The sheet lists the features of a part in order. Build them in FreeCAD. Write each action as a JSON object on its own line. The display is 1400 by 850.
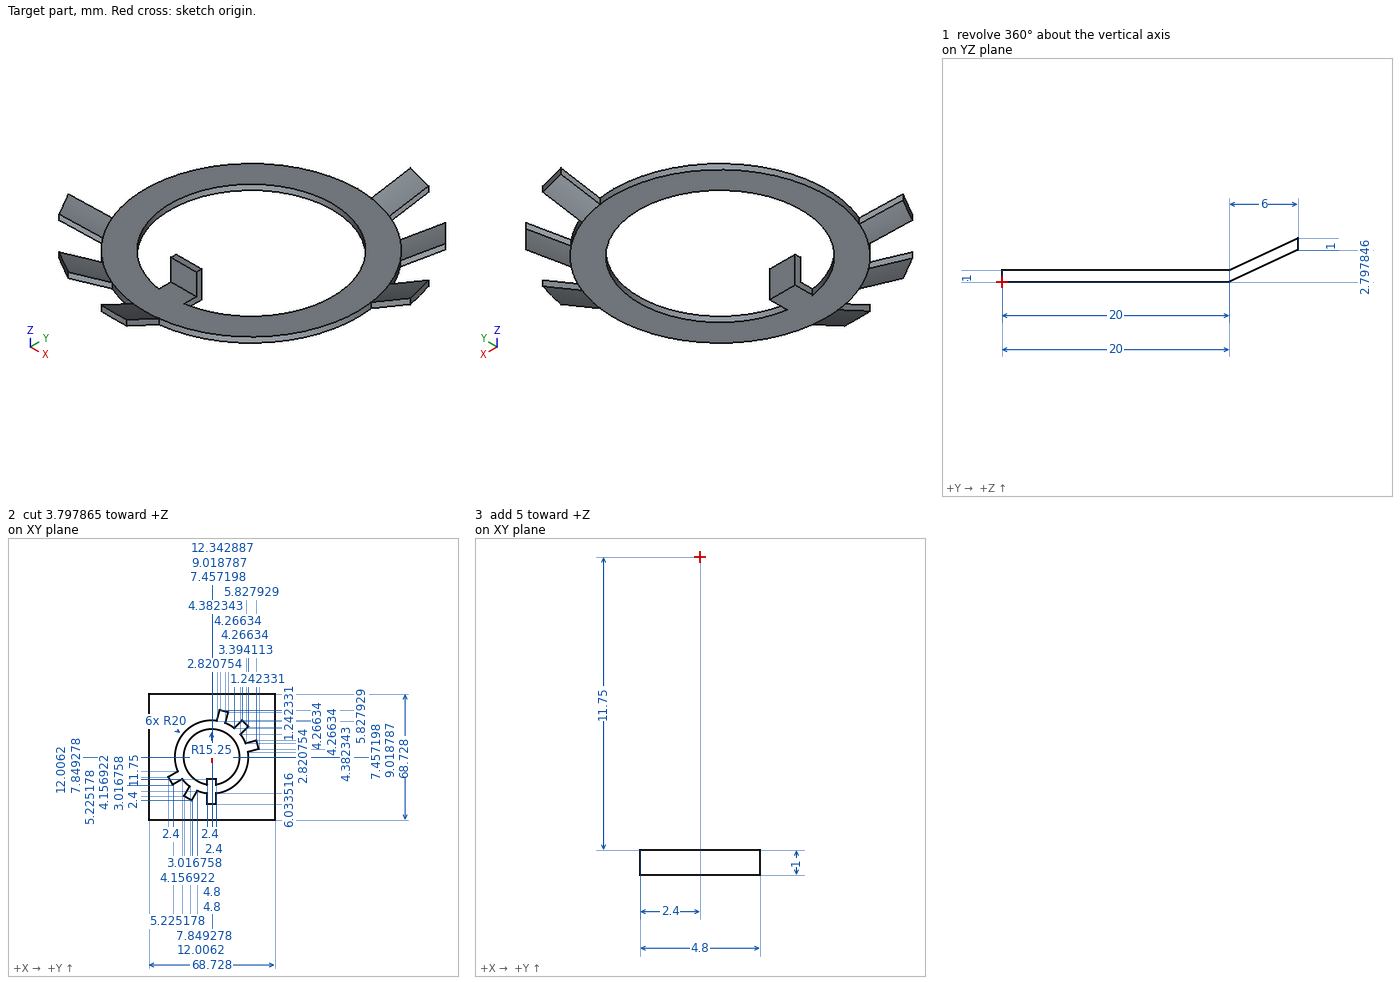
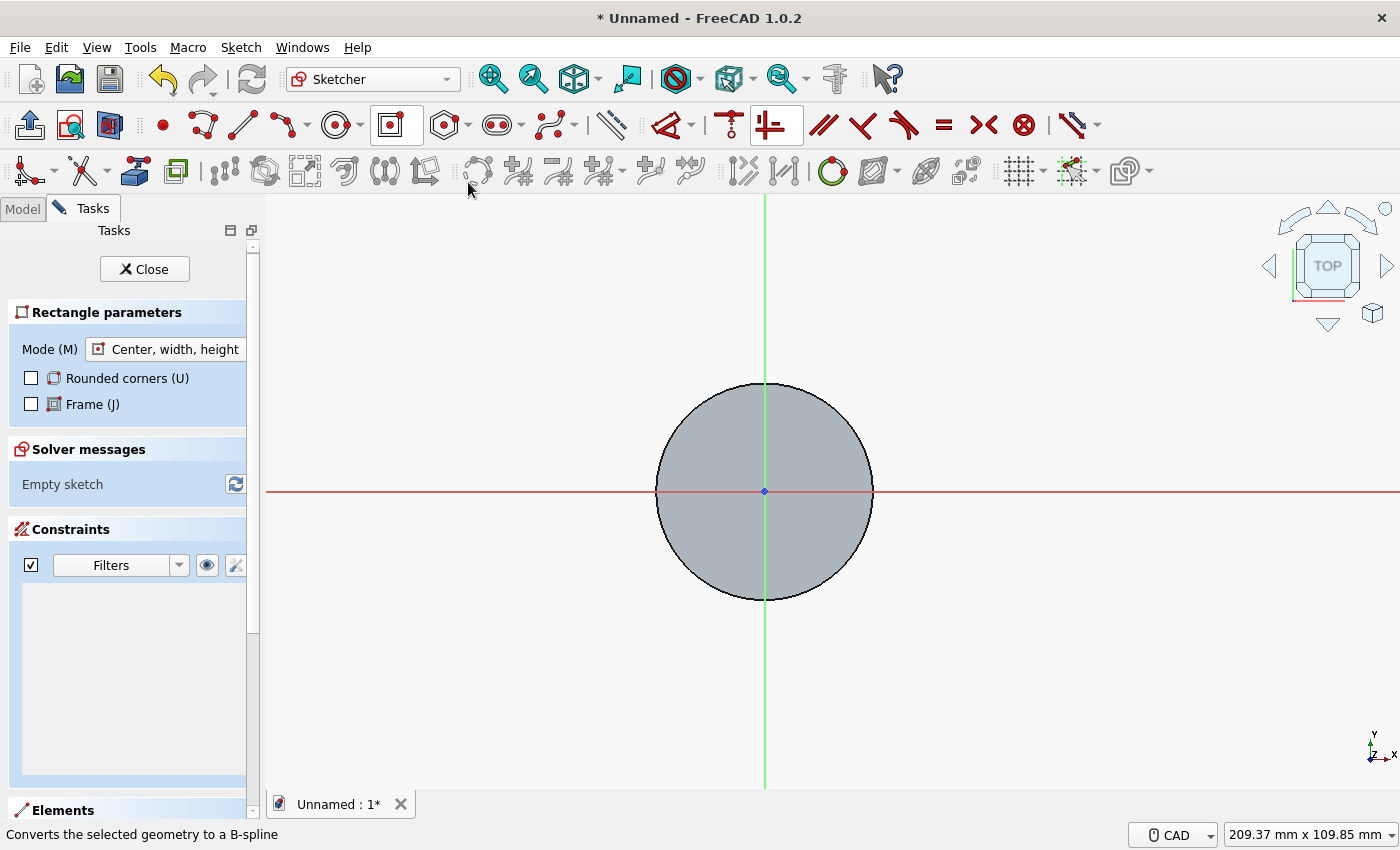
{"action": "left_click", "coordinate": [765, 492]}
{"action": "mouse_move", "coordinate": [951, 306]}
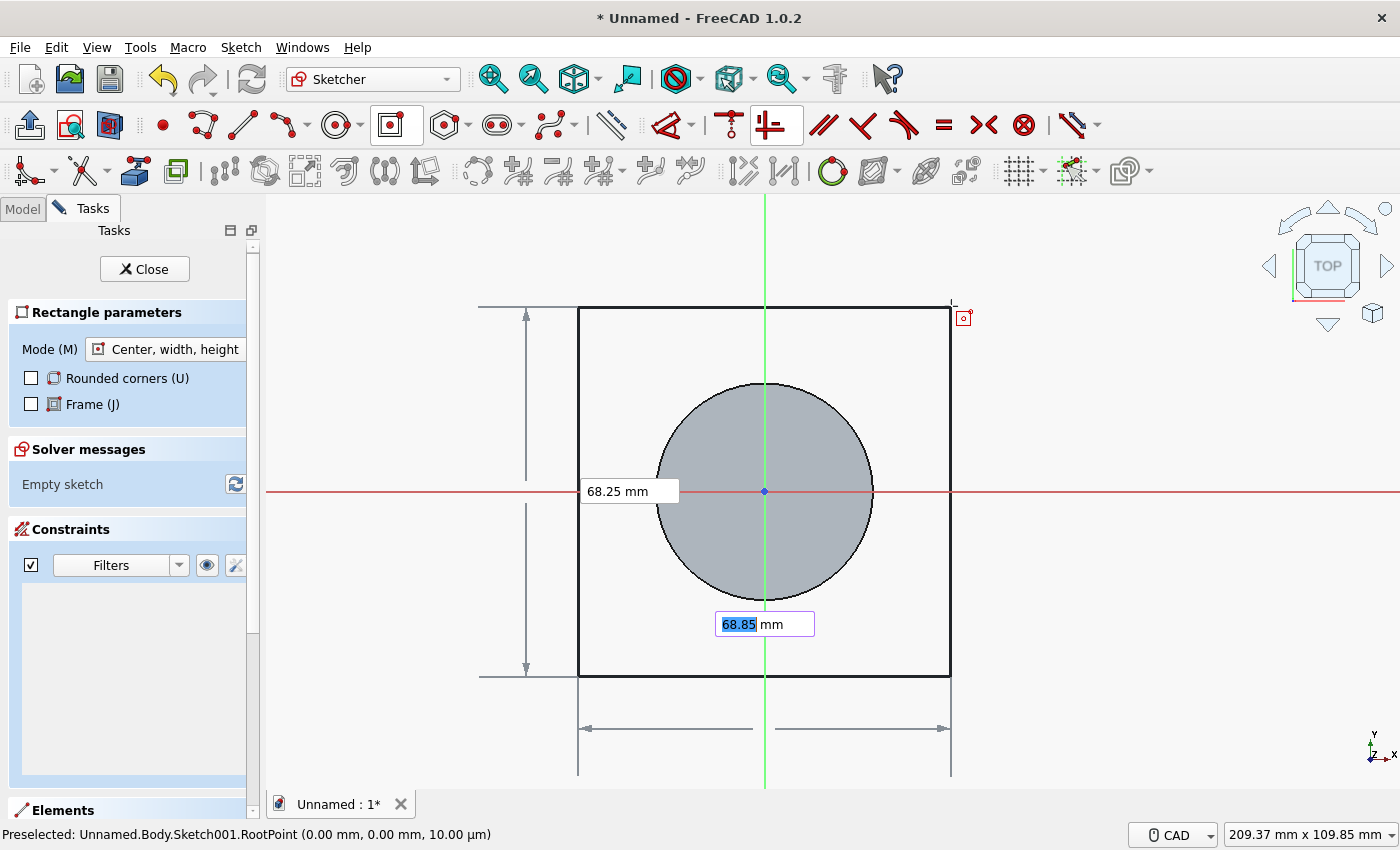
{"action": "type", "text": "68.728"}
{"action": "key", "text": "Tab"}
{"action": "type", "text": "68.728"}
{"action": "key", "text": "Return"}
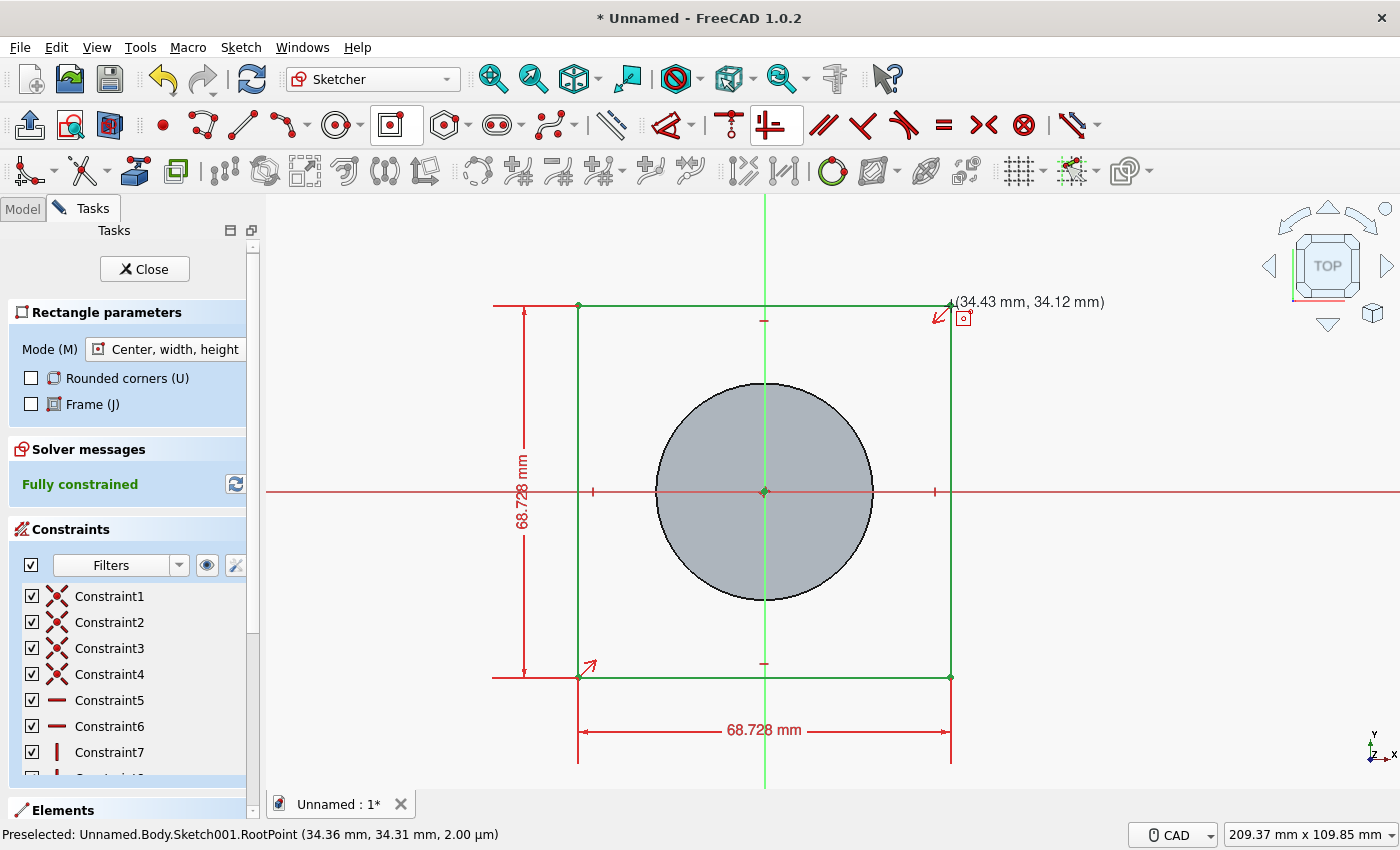
{"action": "left_click", "coordinate": [204, 126]}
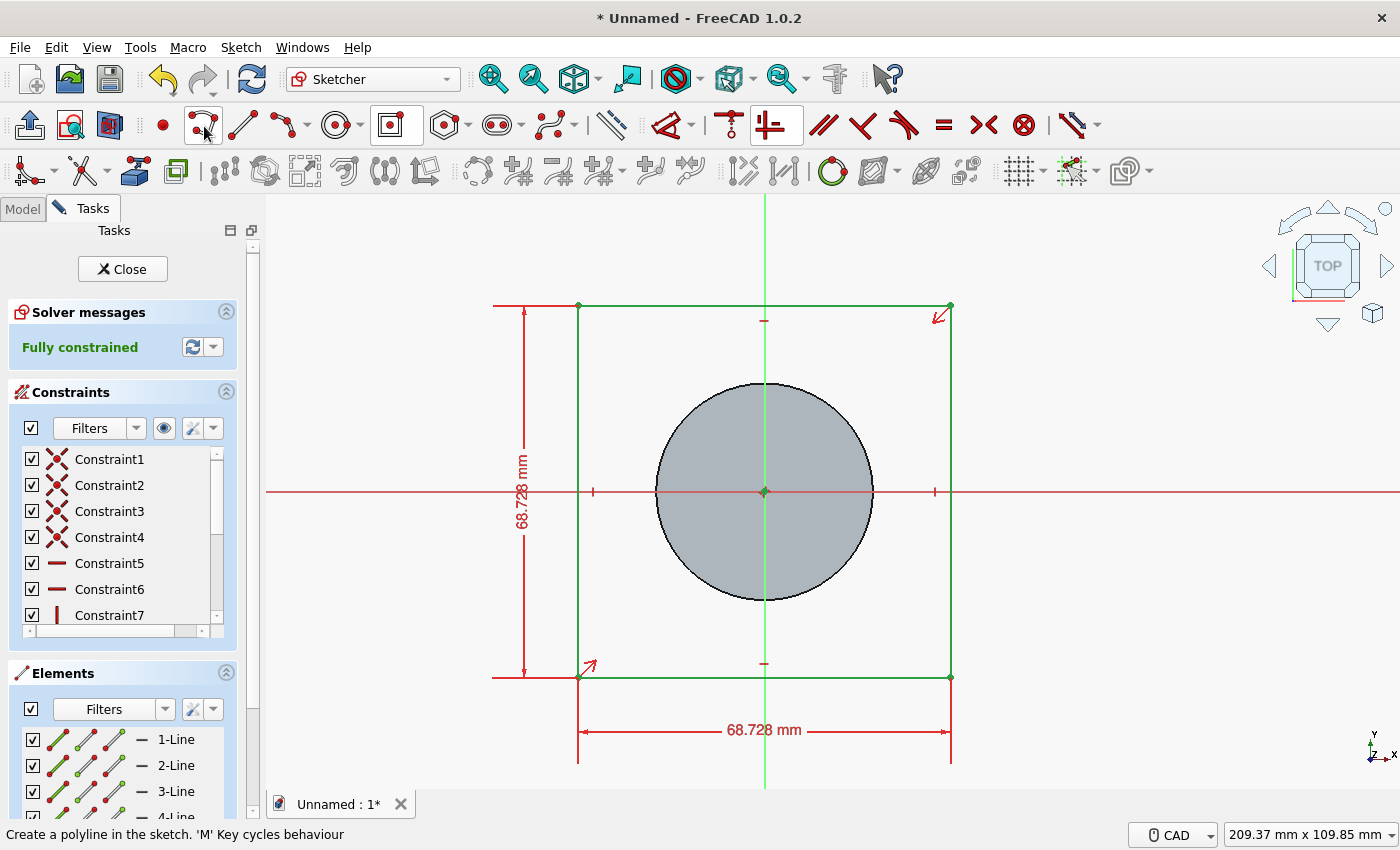
{"action": "scroll", "coordinate": [752, 573], "scroll_direction": "up", "scroll_amount": 2}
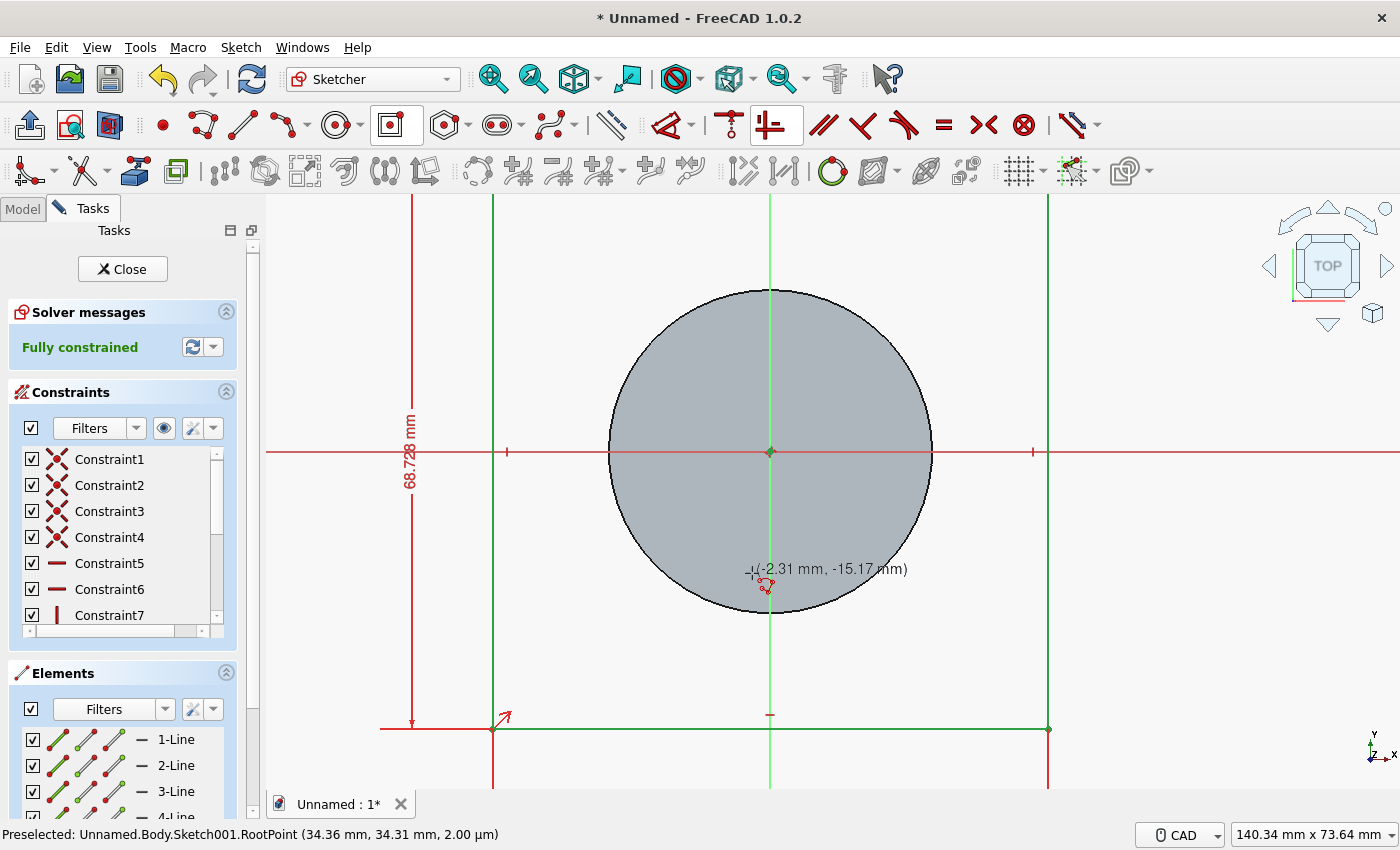
{"action": "left_click", "coordinate": [751, 573]}
{"action": "left_click", "coordinate": [751, 547]}
{"action": "left_click", "coordinate": [790, 547]}
{"action": "left_click", "coordinate": [790, 573]}
{"action": "right_click", "coordinate": [790, 573]}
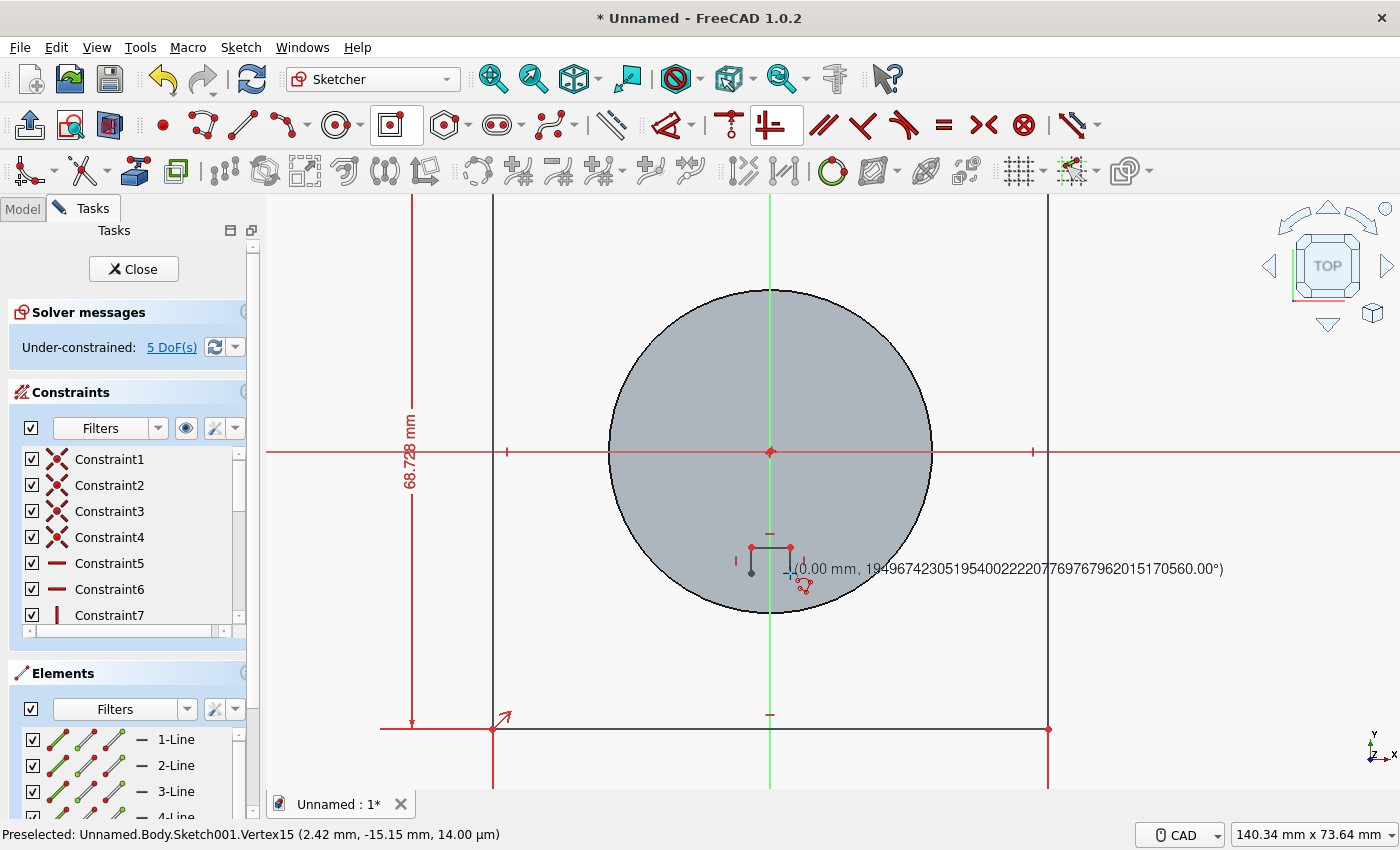
{"action": "left_click", "coordinate": [284, 126]}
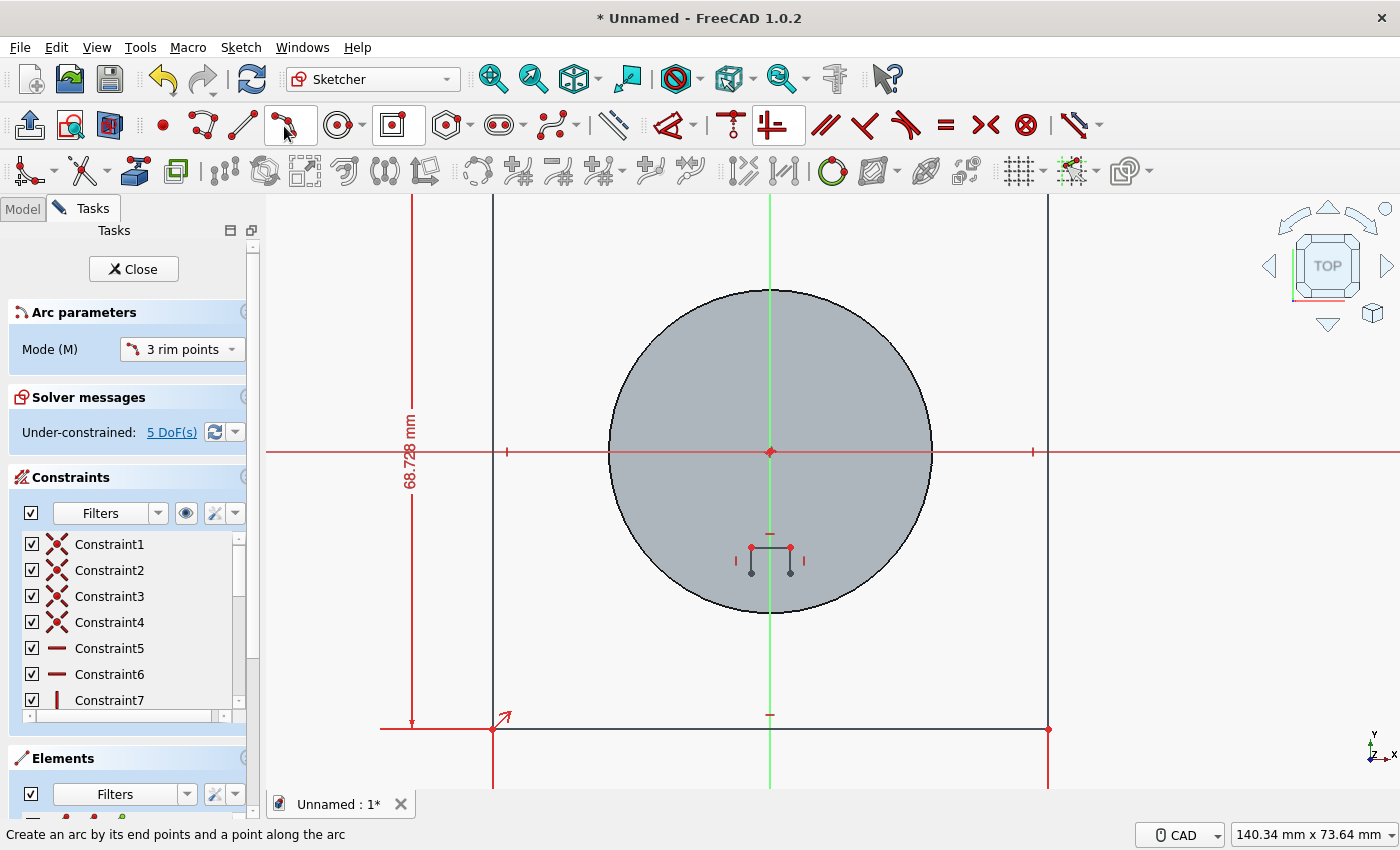
{"action": "left_click", "coordinate": [790, 574]}
{"action": "left_click", "coordinate": [751, 574]}
{"action": "left_click", "coordinate": [840, 350]}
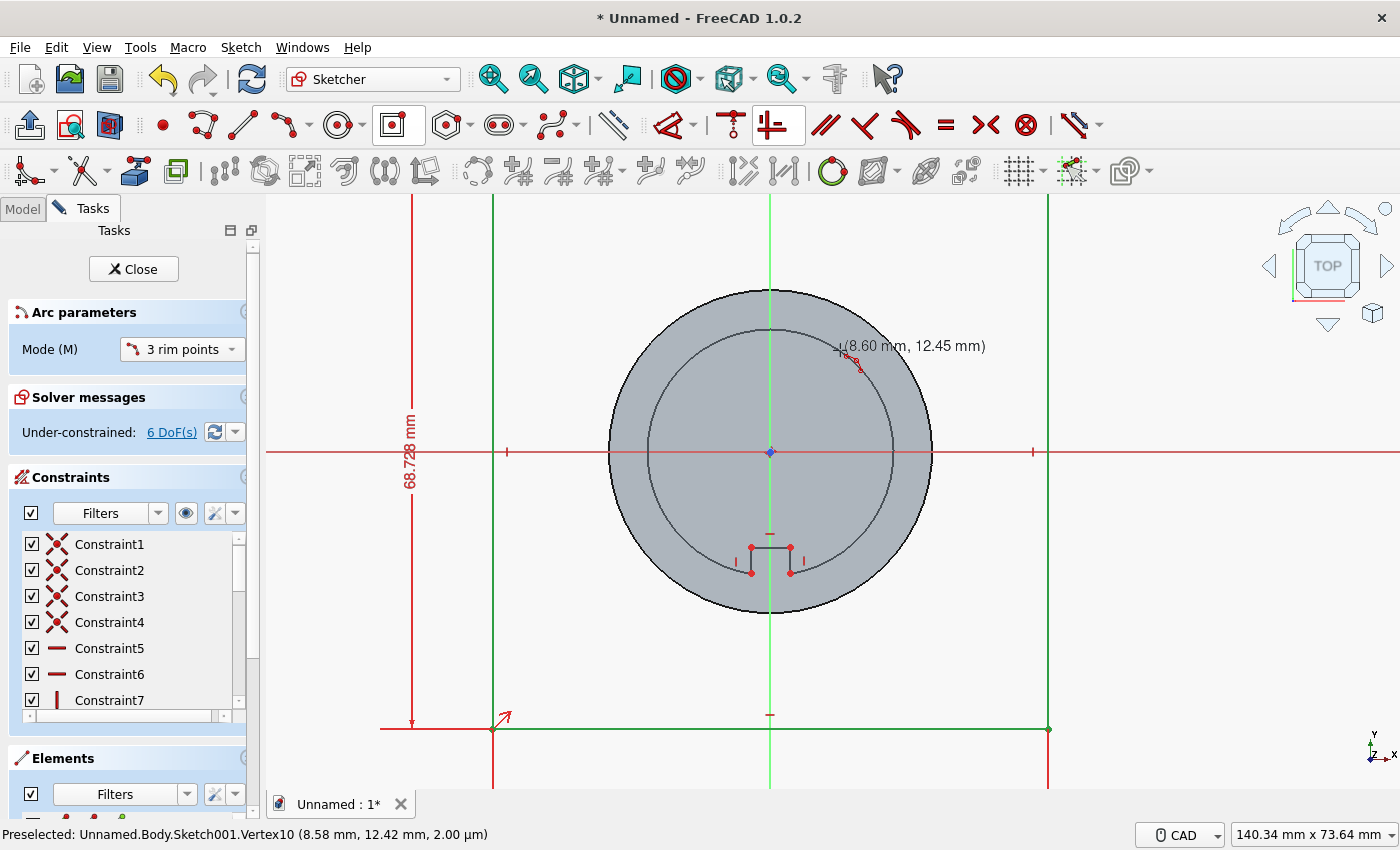
{"action": "left_click", "coordinate": [204, 126]}